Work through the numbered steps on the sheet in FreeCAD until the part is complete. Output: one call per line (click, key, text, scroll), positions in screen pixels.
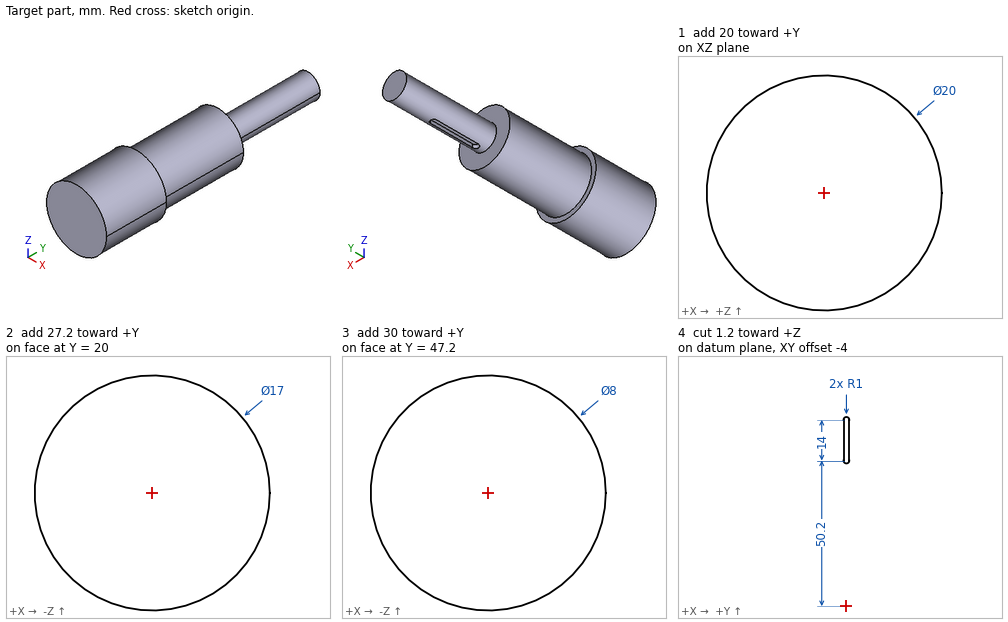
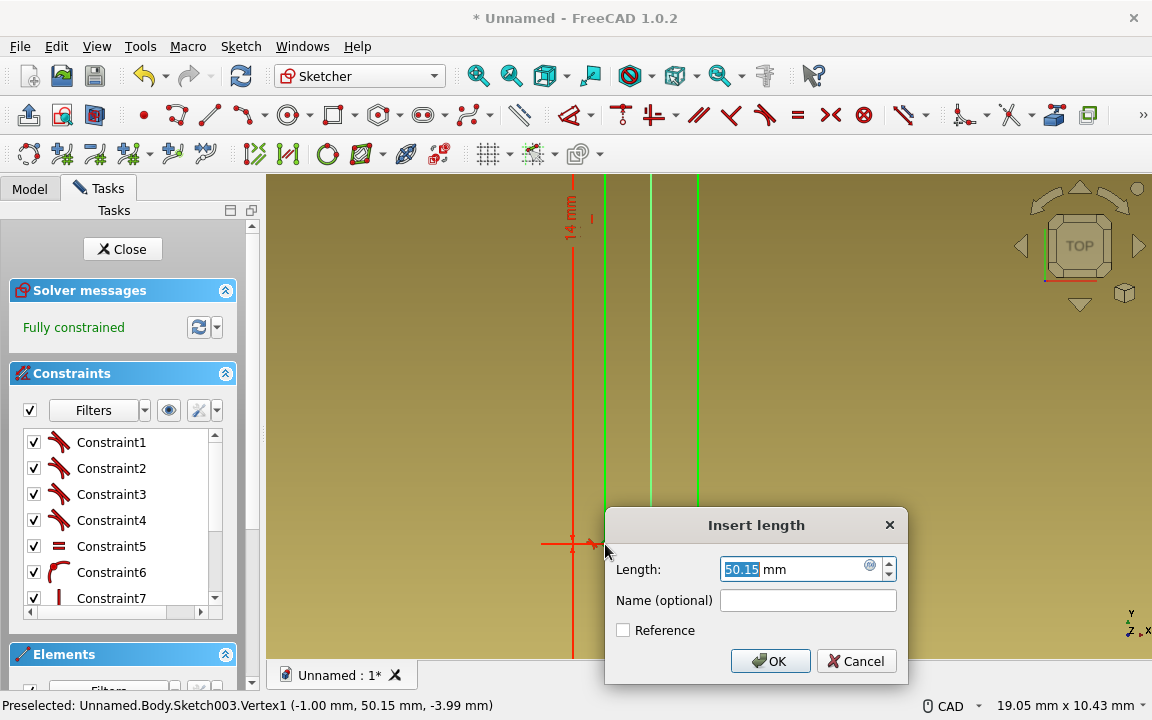
text(50.2)
key(Return)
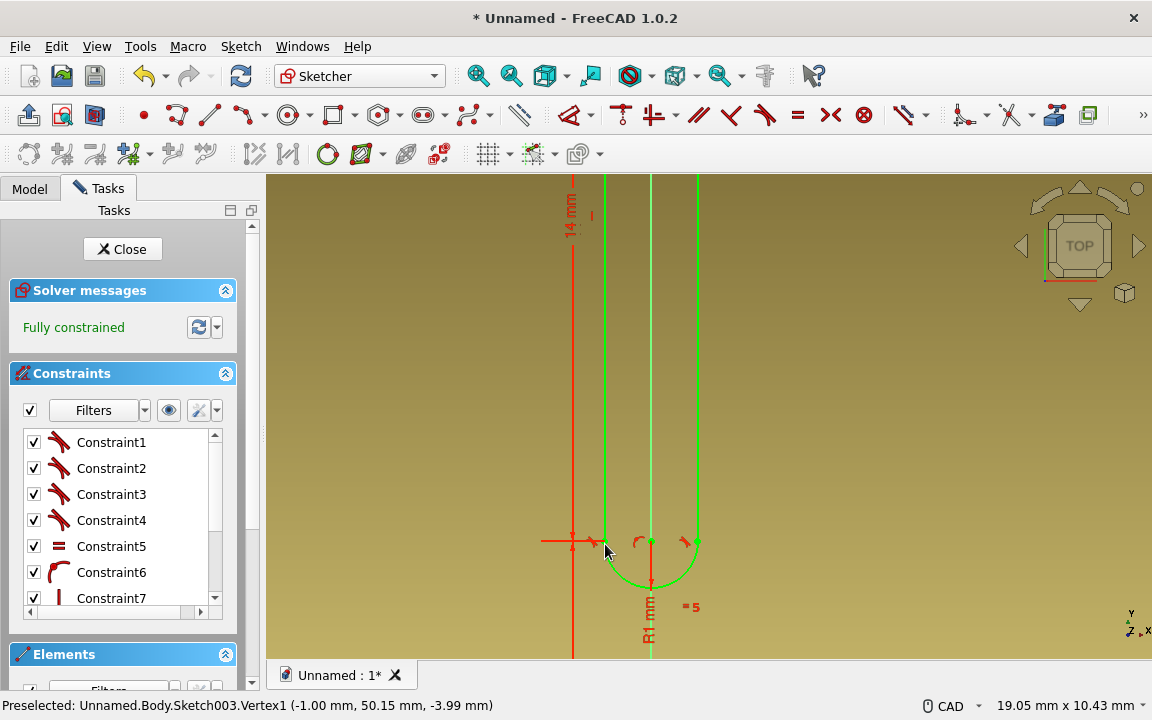
click(123, 249)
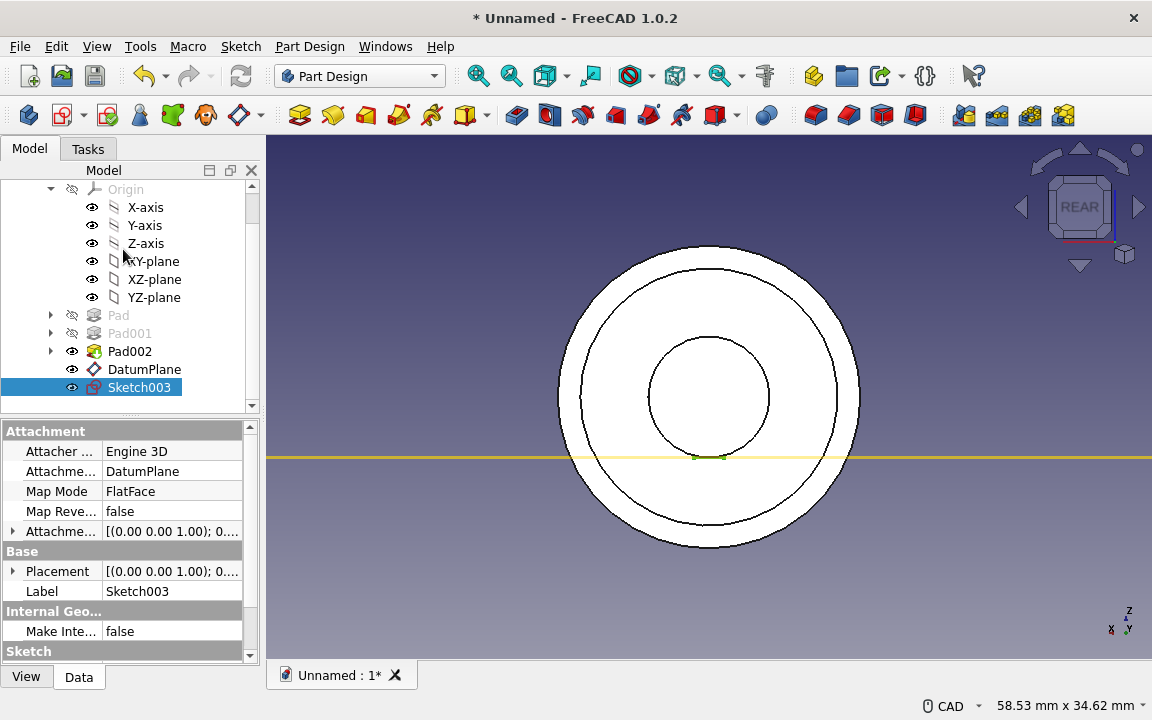
click(517, 116)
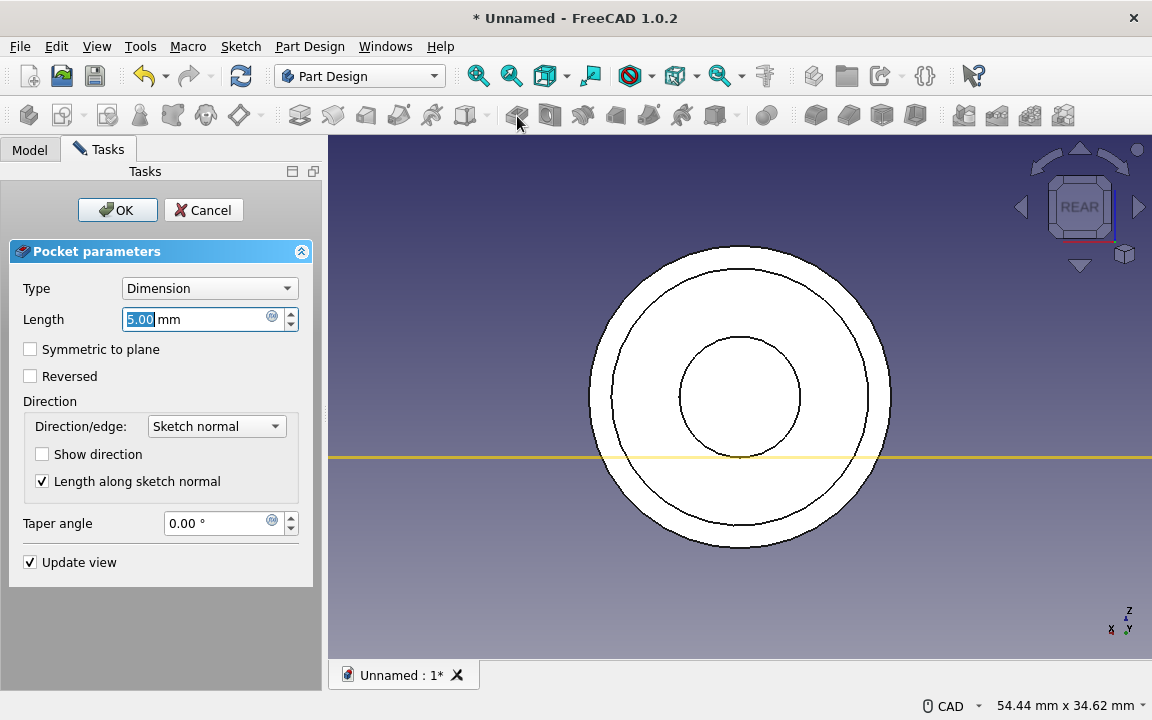
text(1.2)
key(Tab)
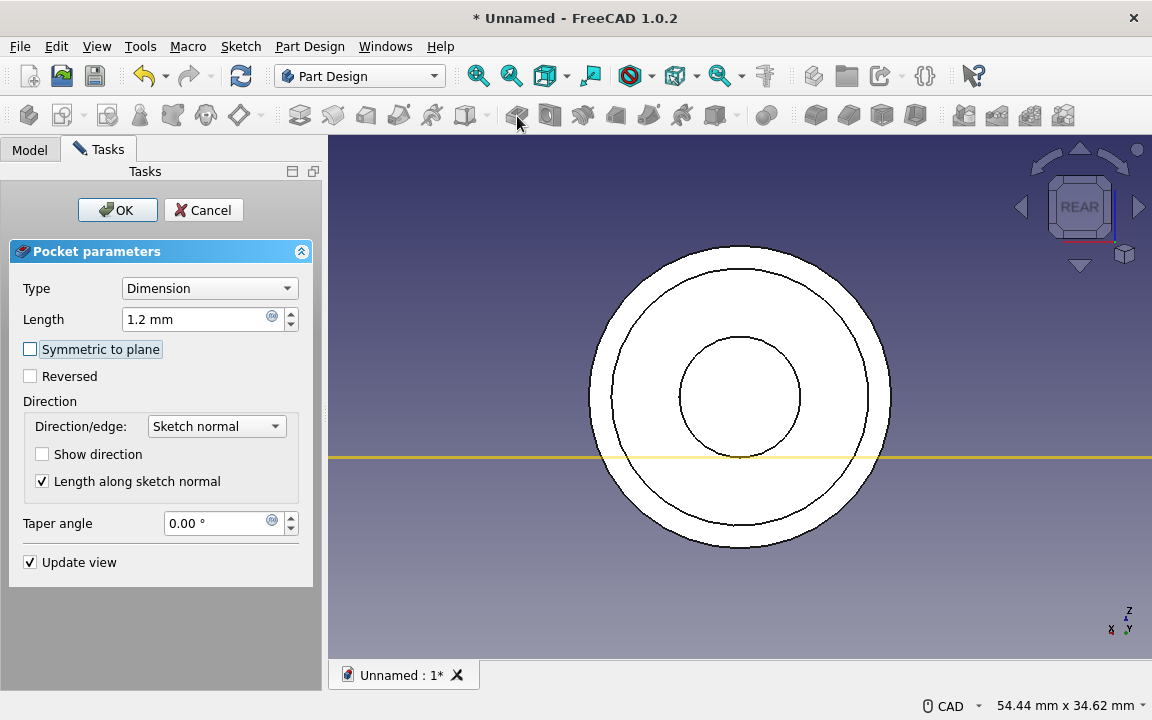
click(31, 376)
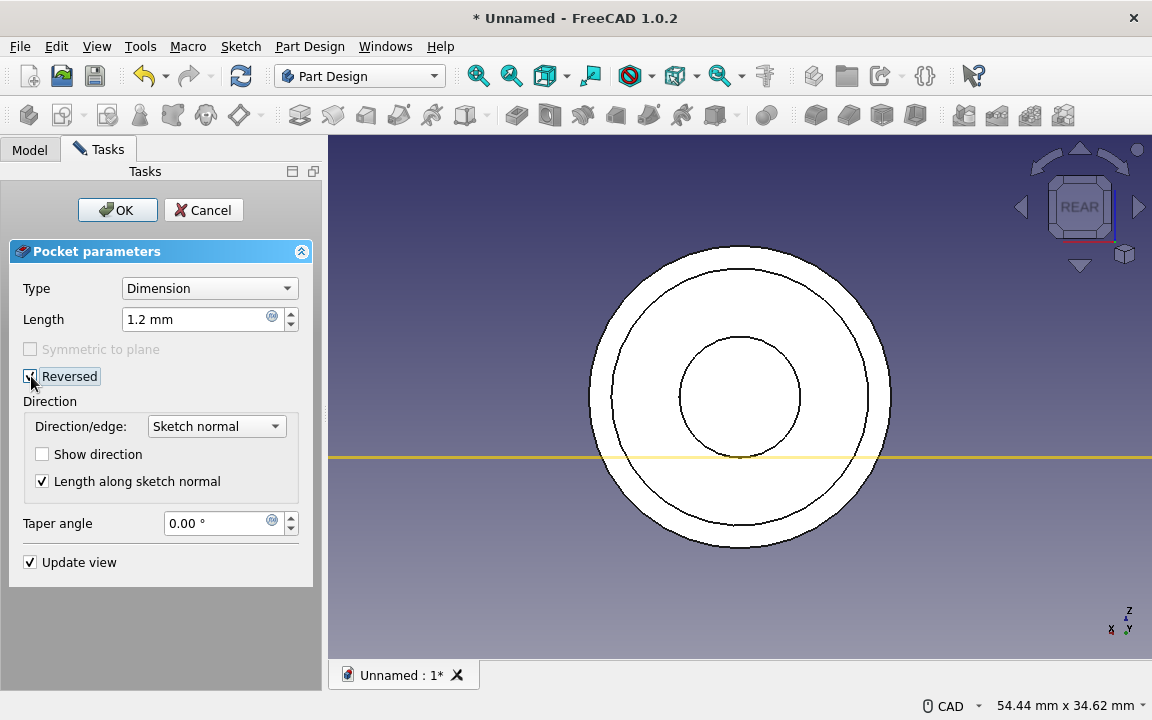
click(118, 210)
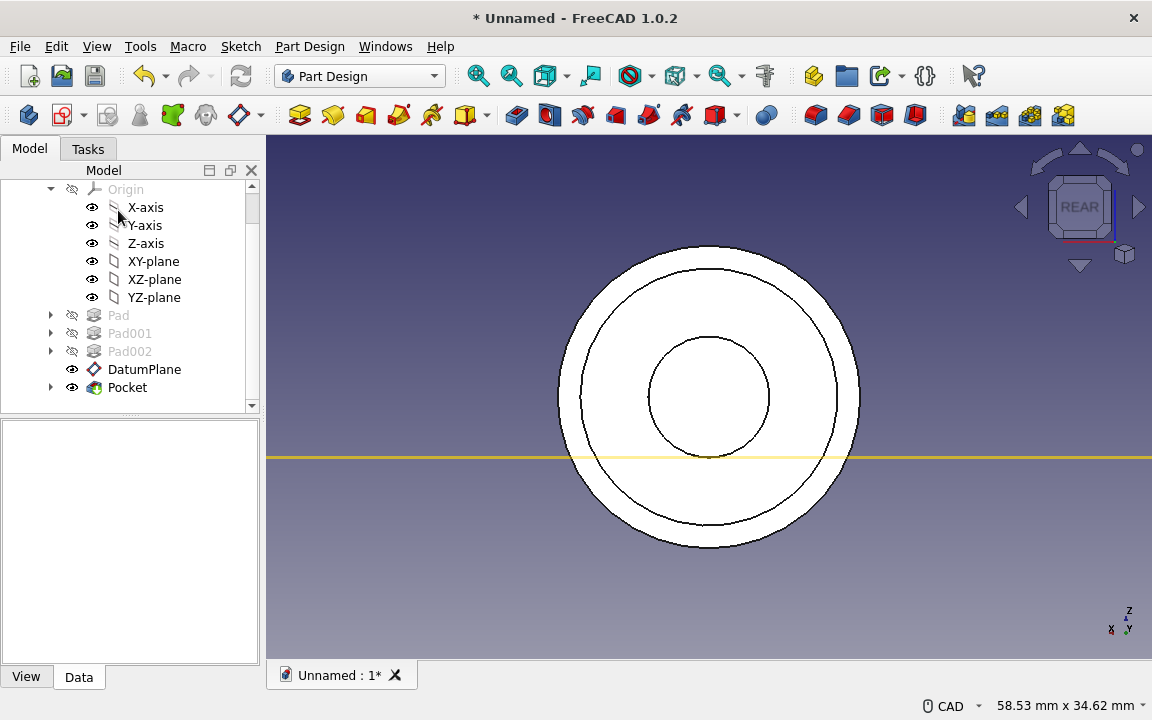
click(117, 369)
key(space)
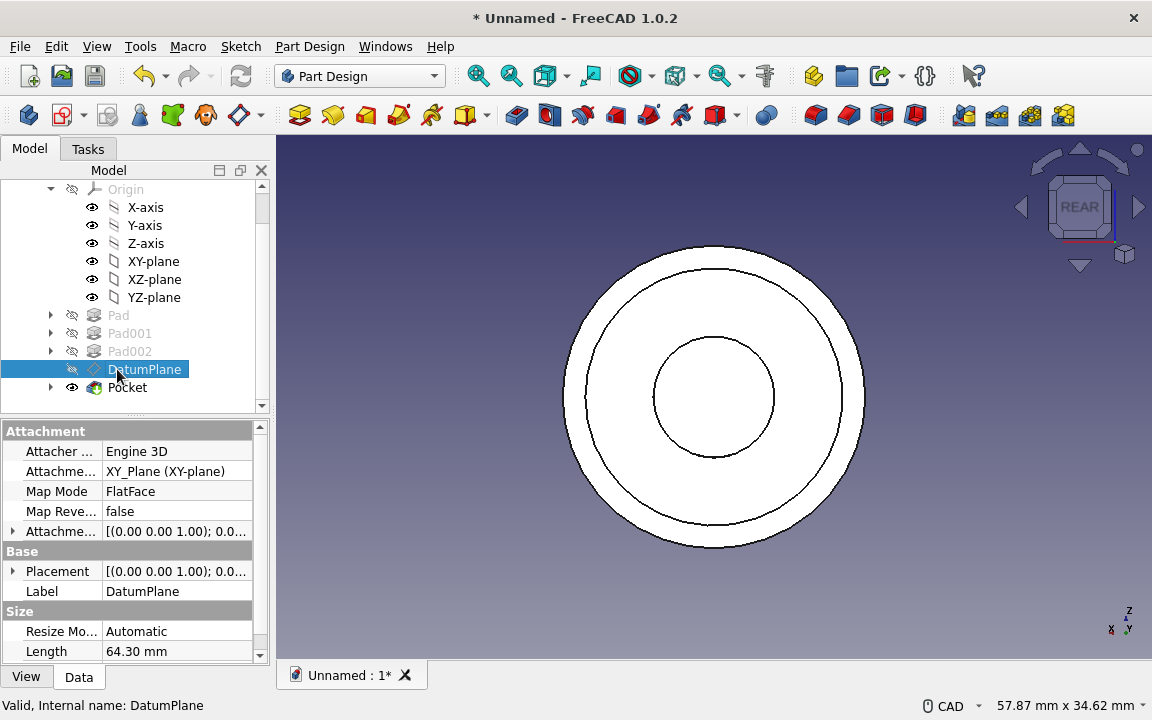
key(0)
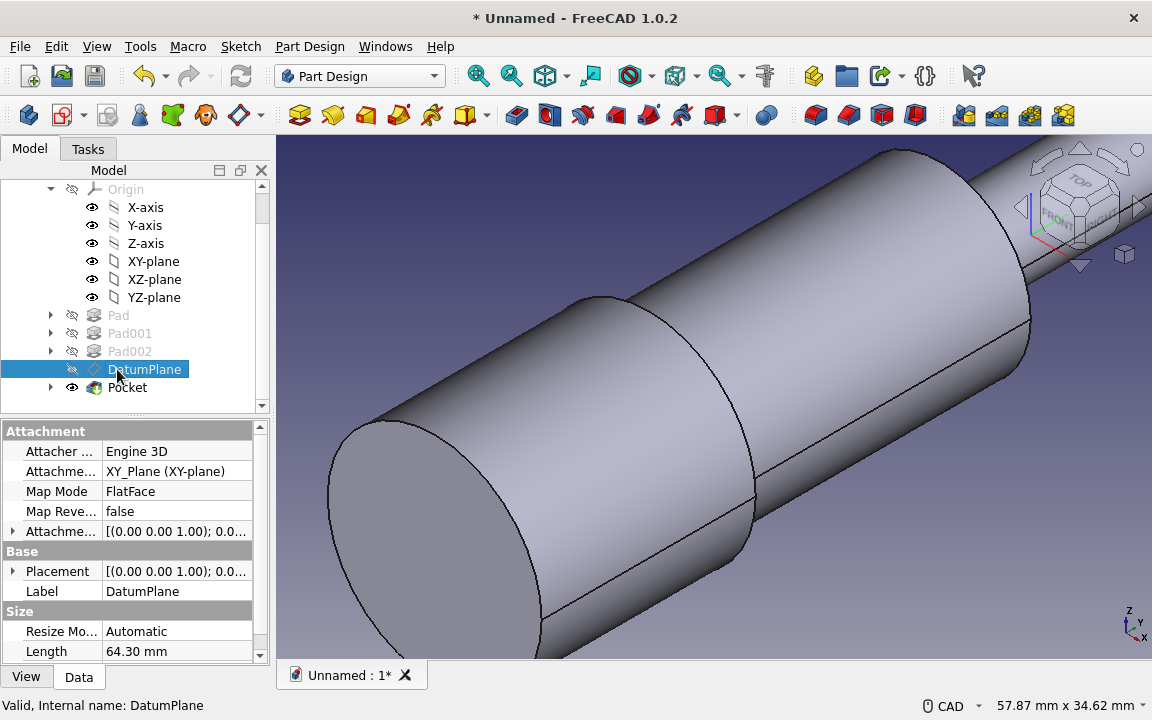
click(479, 76)